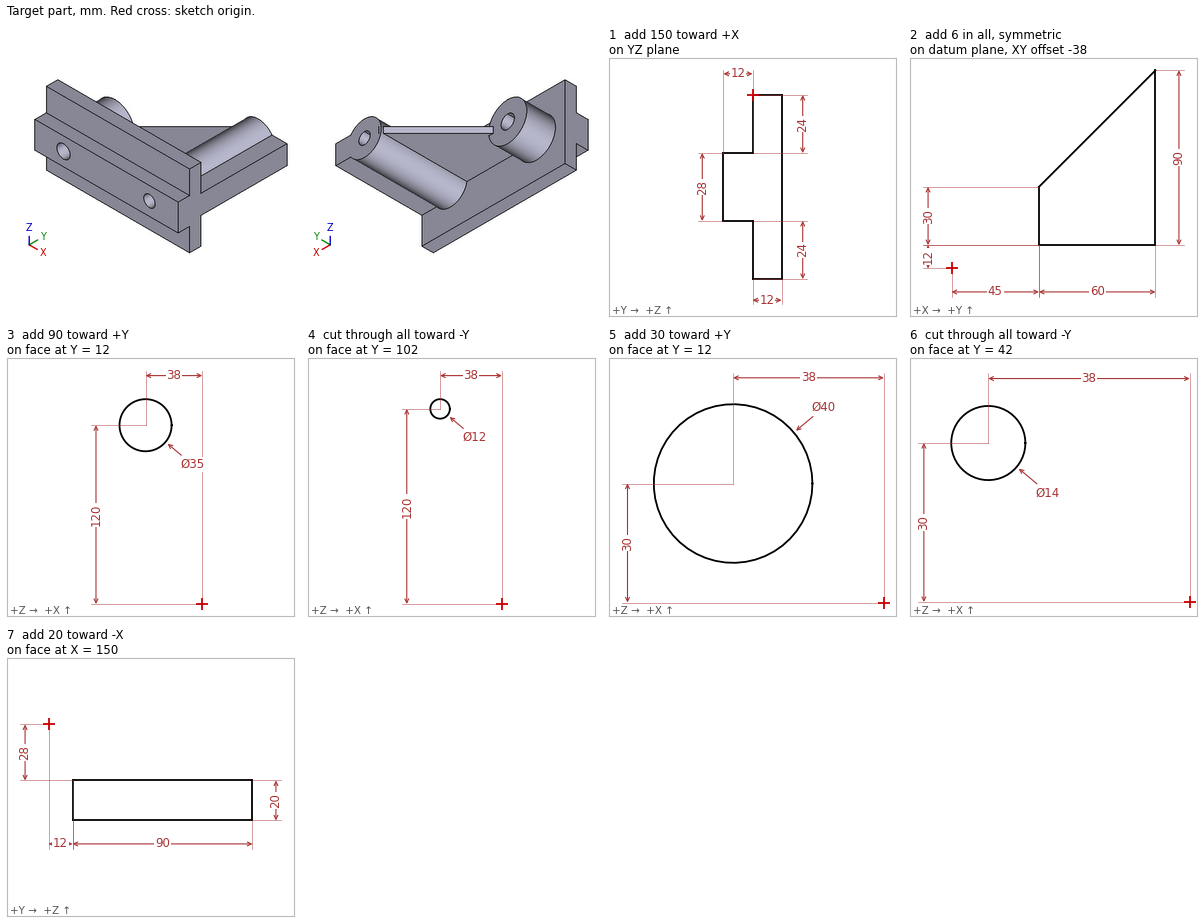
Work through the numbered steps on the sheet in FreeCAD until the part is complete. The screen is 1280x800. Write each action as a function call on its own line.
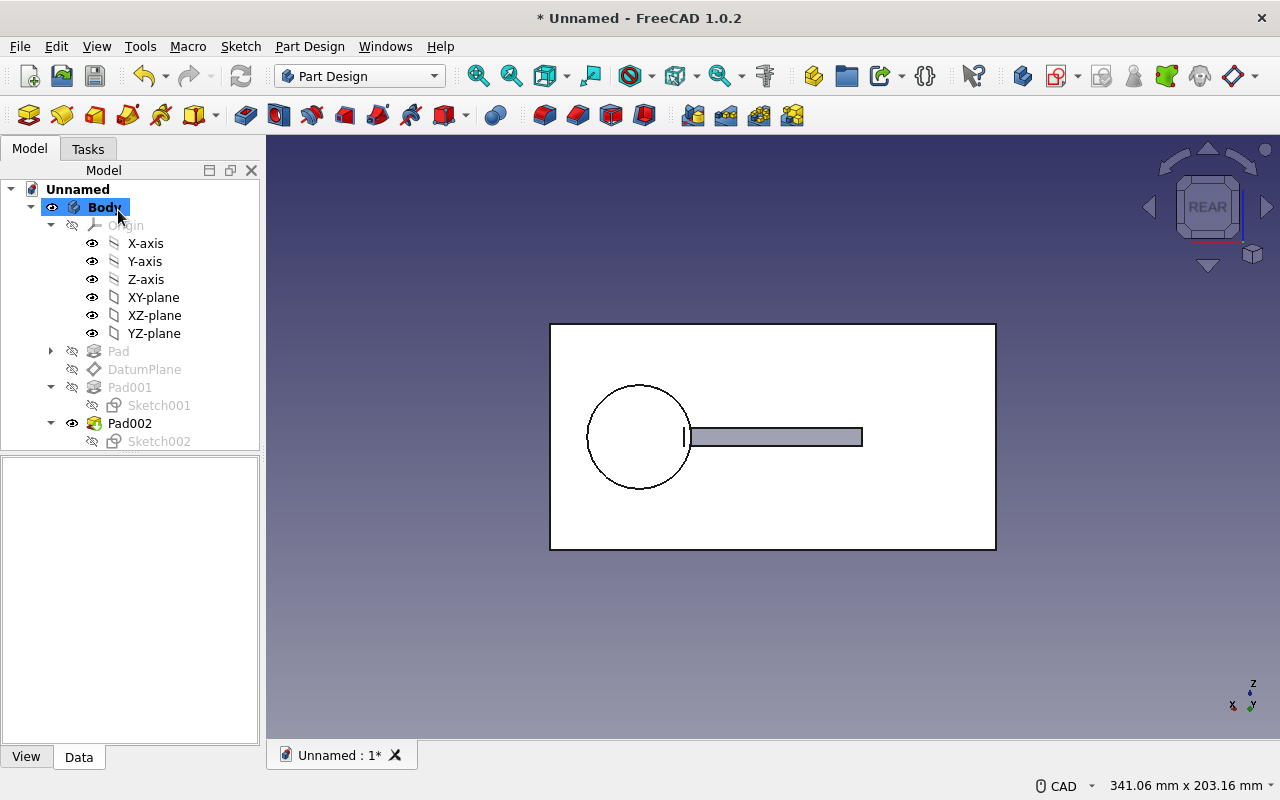
click(479, 76)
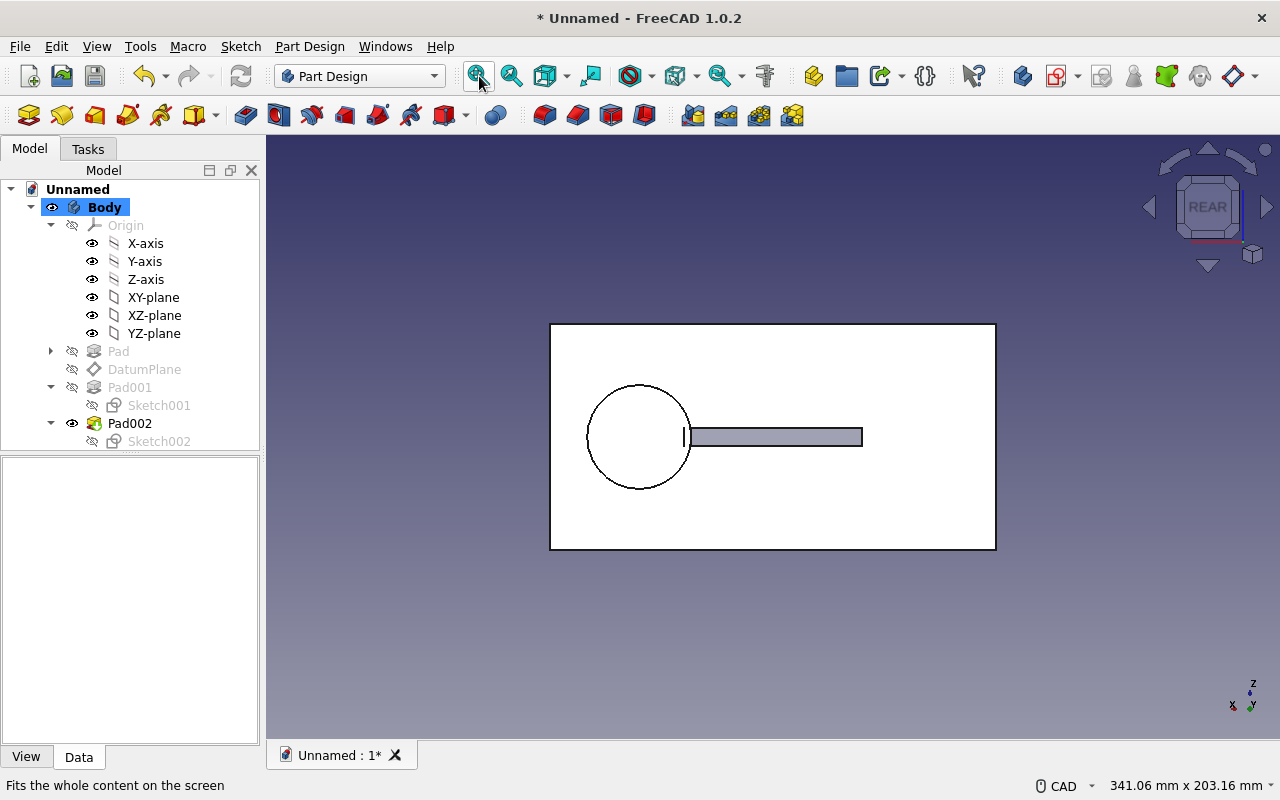
click(639, 436)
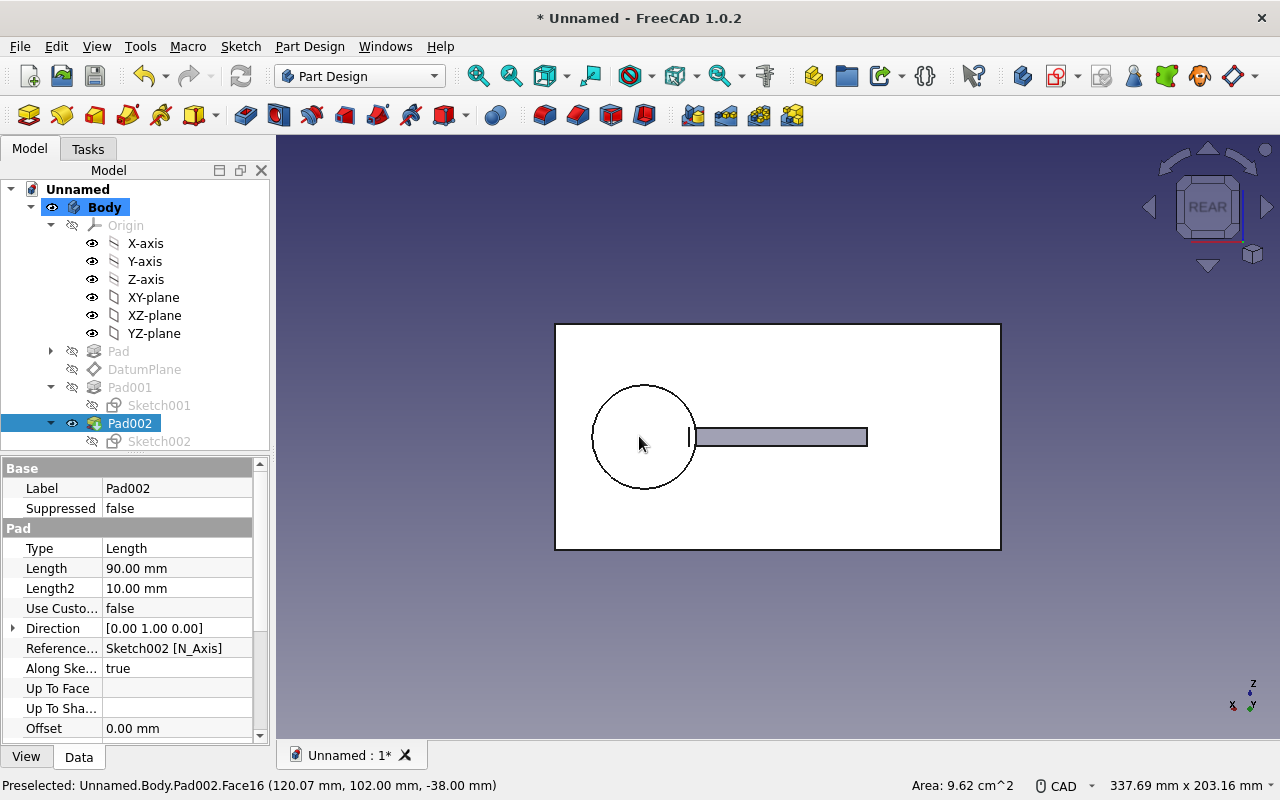
click(1056, 76)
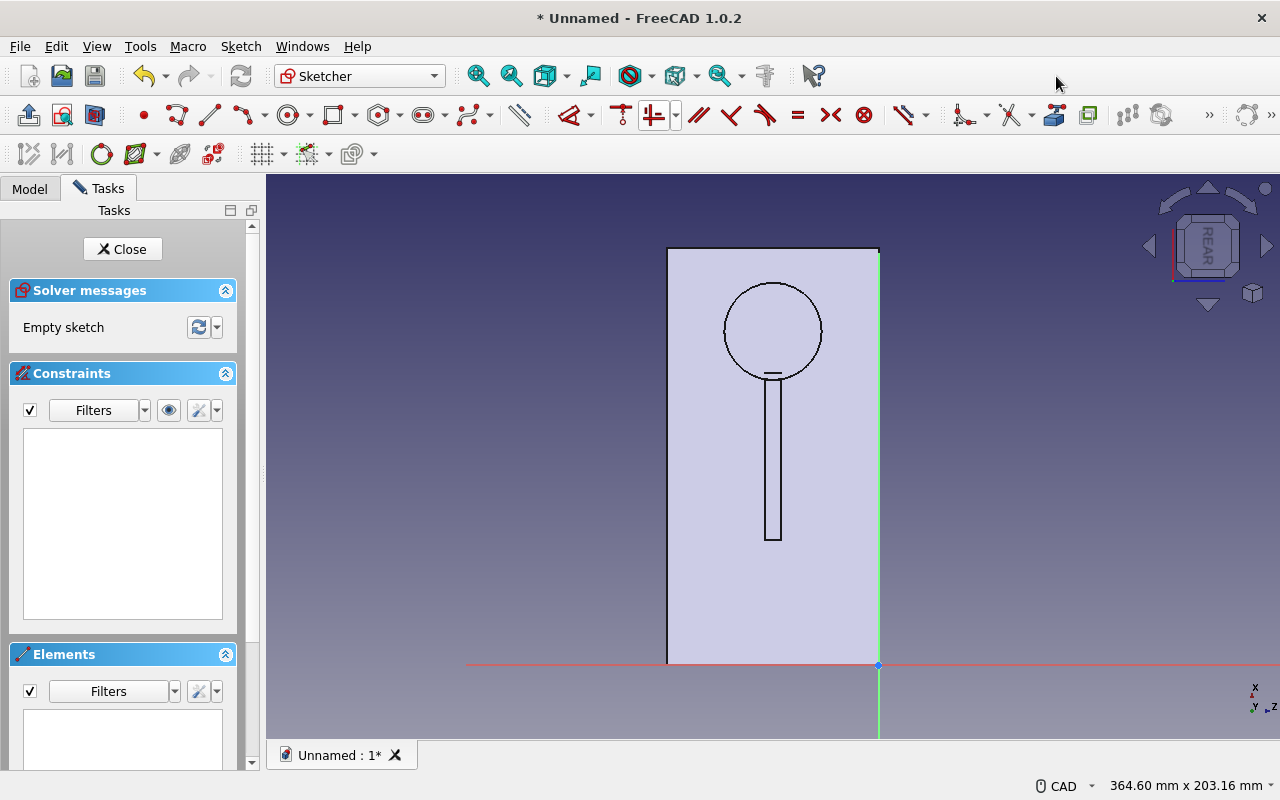
scroll(780, 319, up, 12)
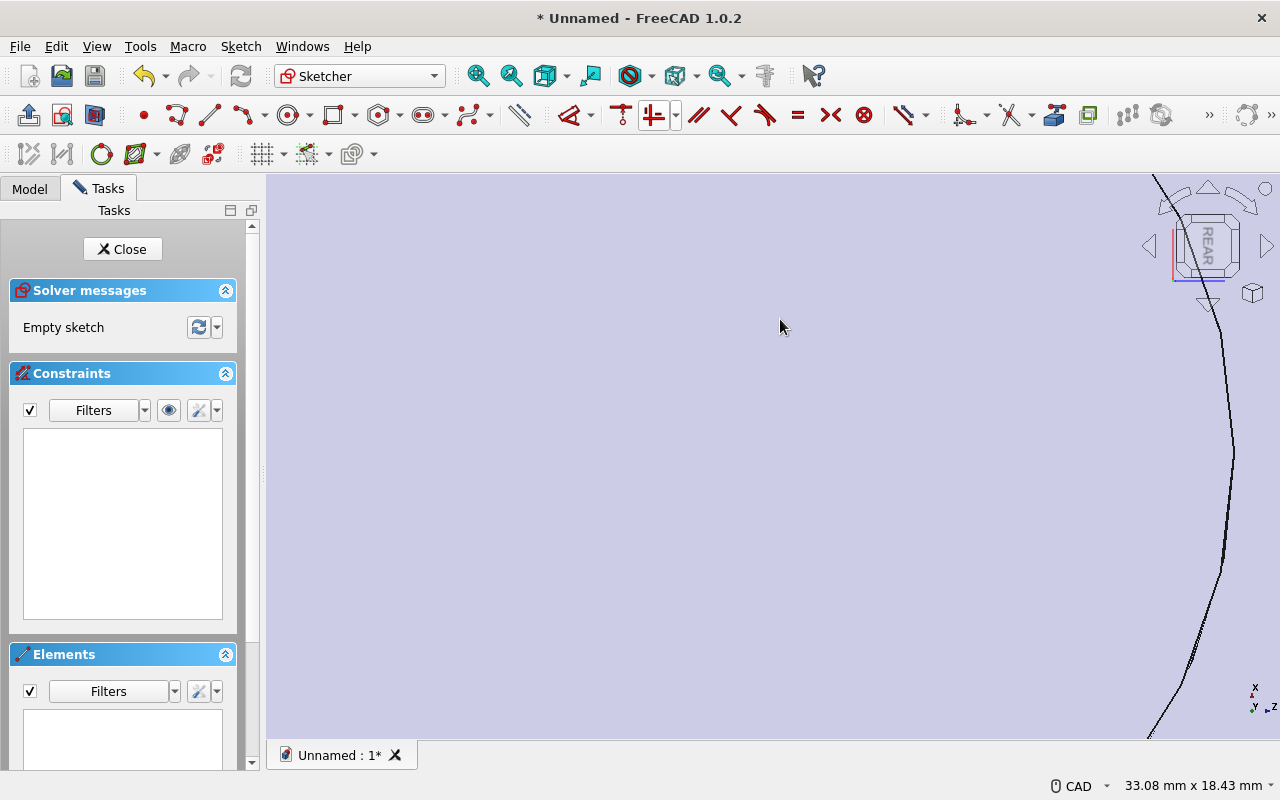
click(288, 116)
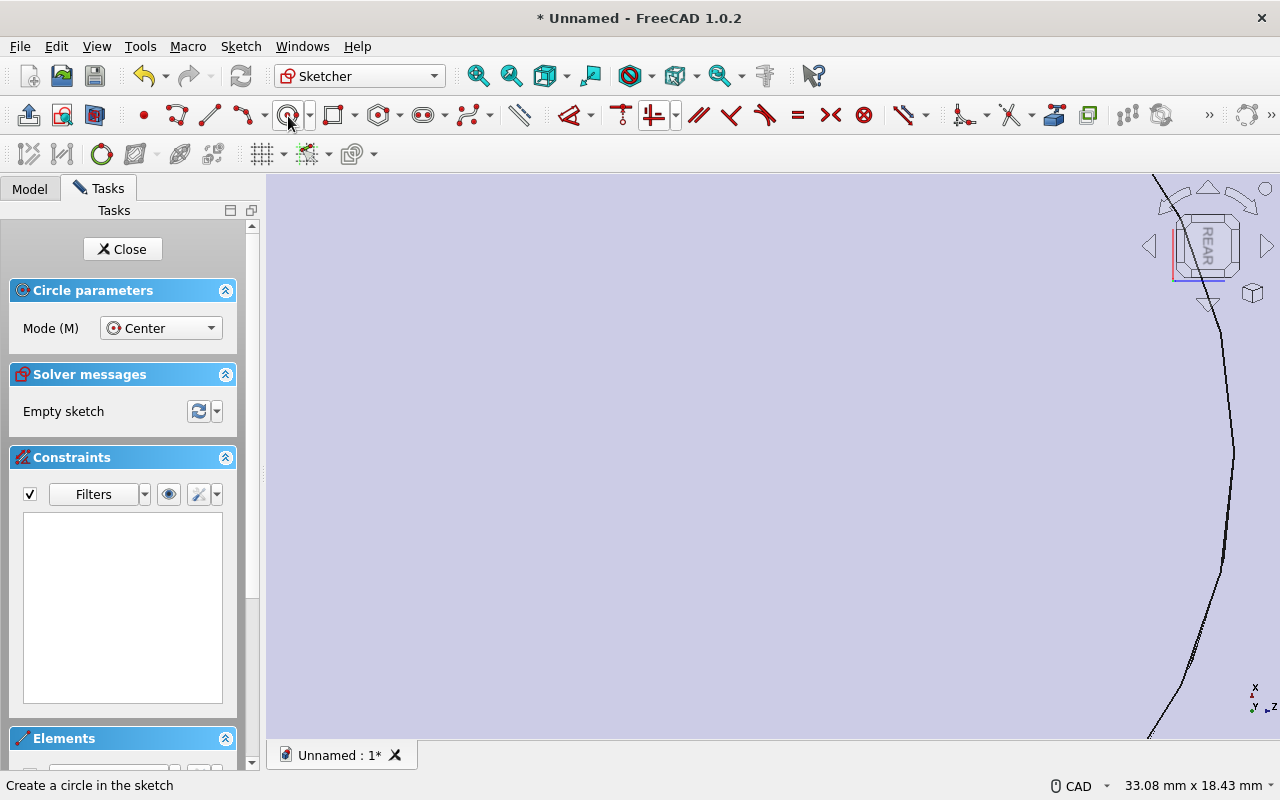
click(698, 453)
move(828, 322)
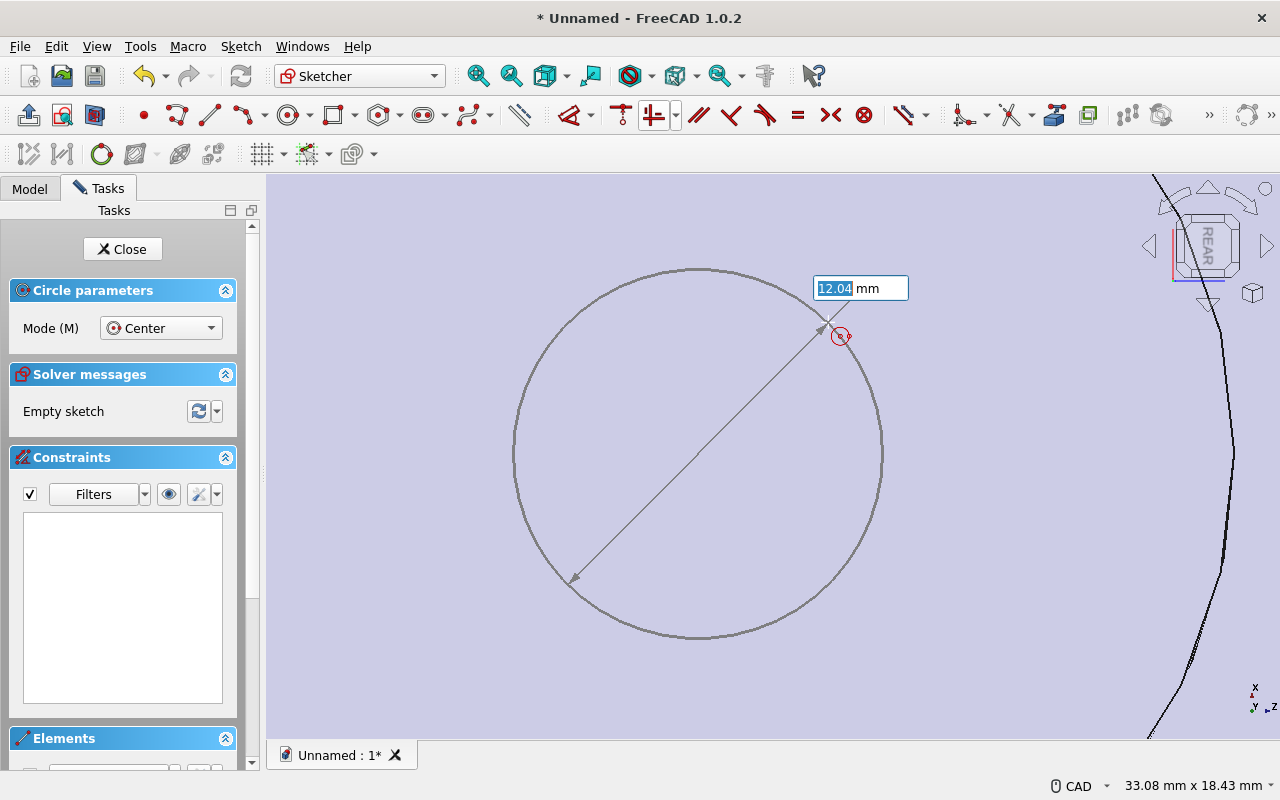
text(12)
key(Return)
key(Escape)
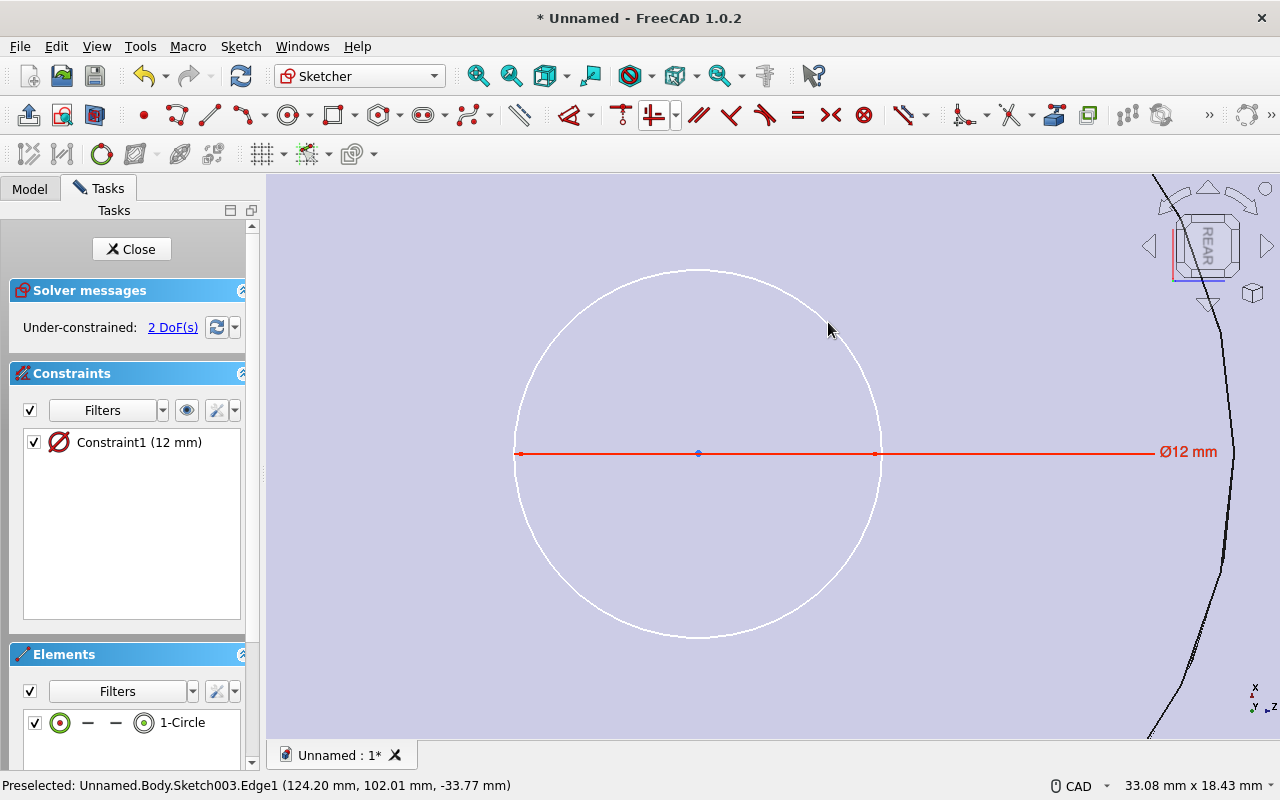
click(568, 116)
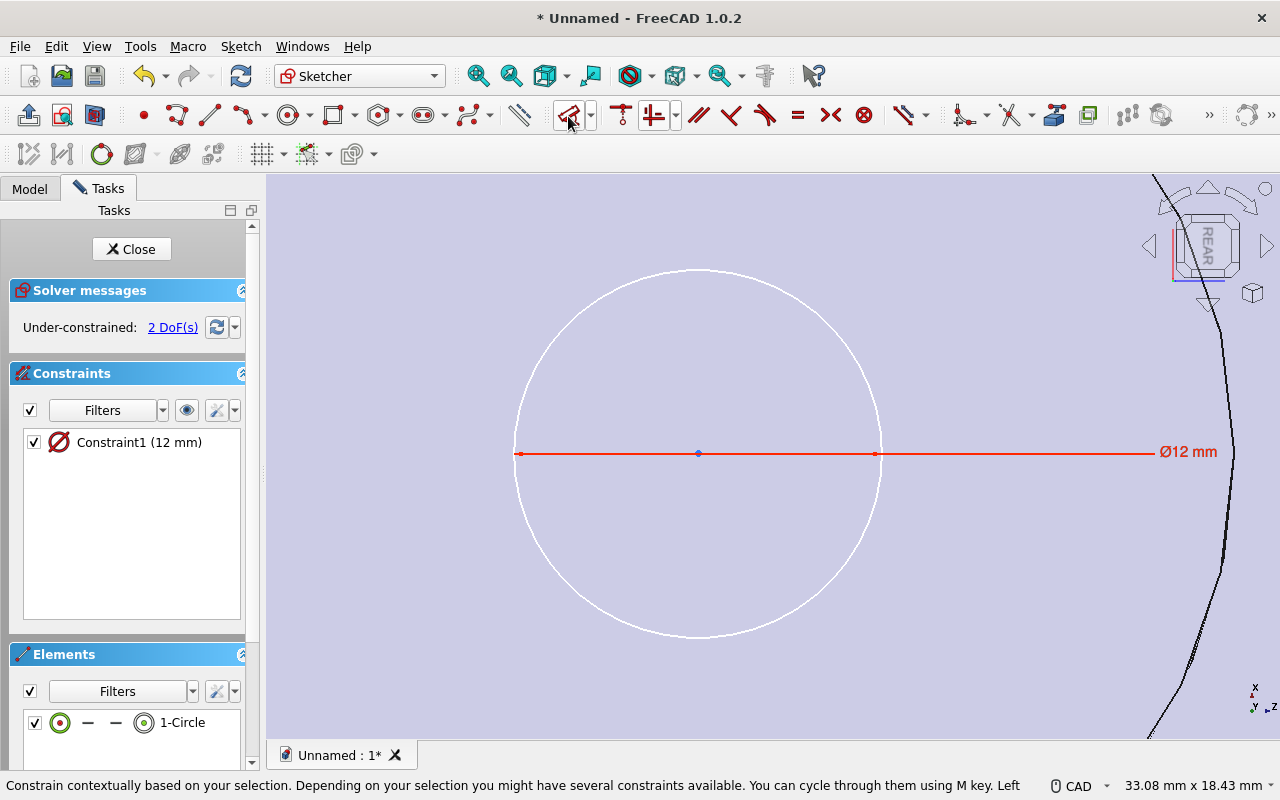
click(698, 454)
click(906, 420)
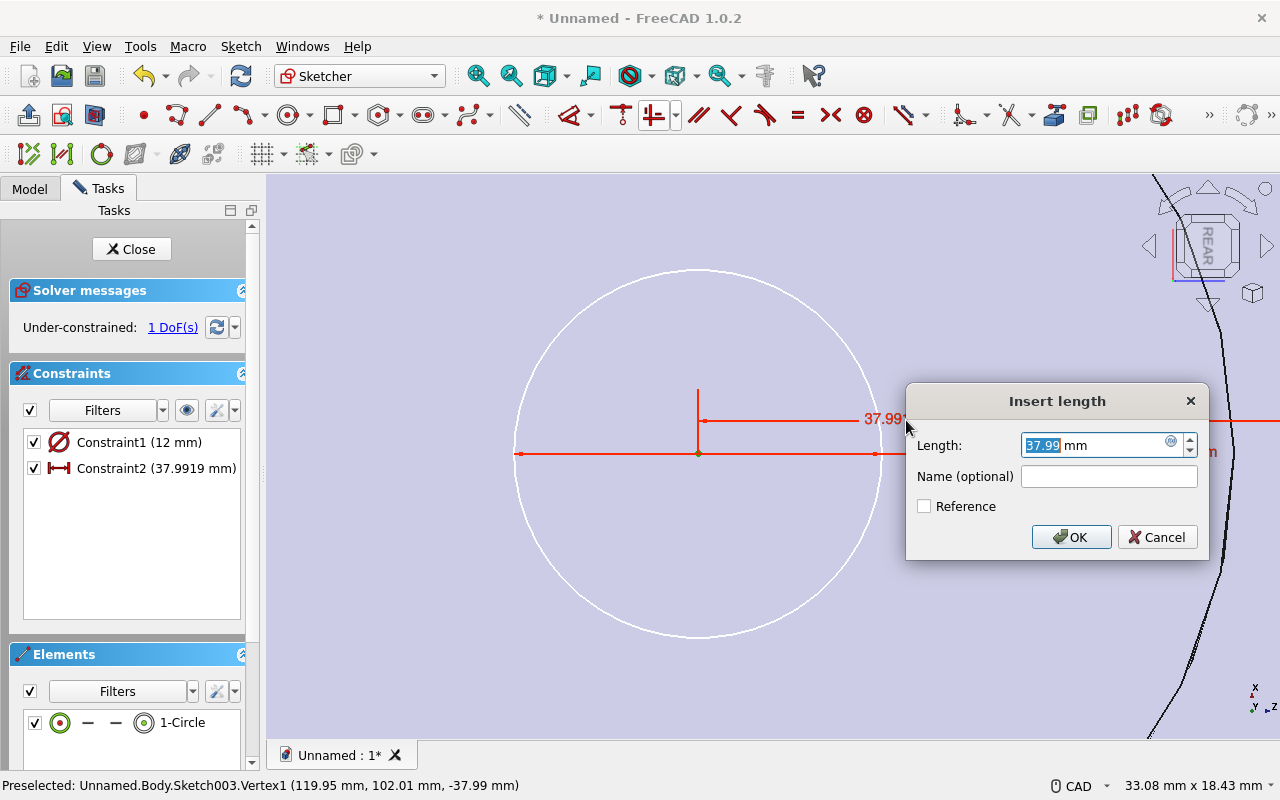
text(38)
key(Return)